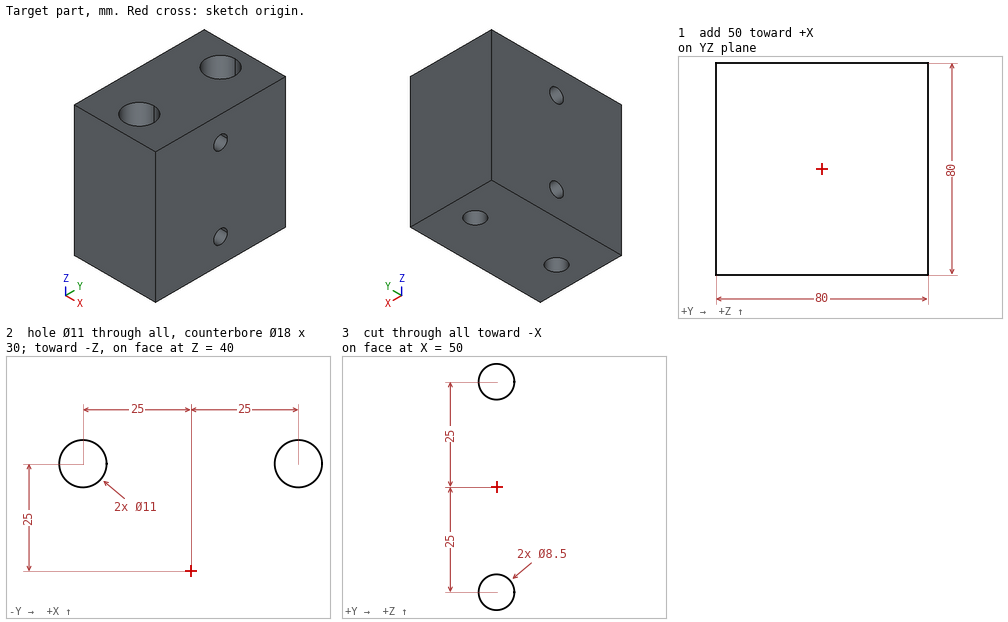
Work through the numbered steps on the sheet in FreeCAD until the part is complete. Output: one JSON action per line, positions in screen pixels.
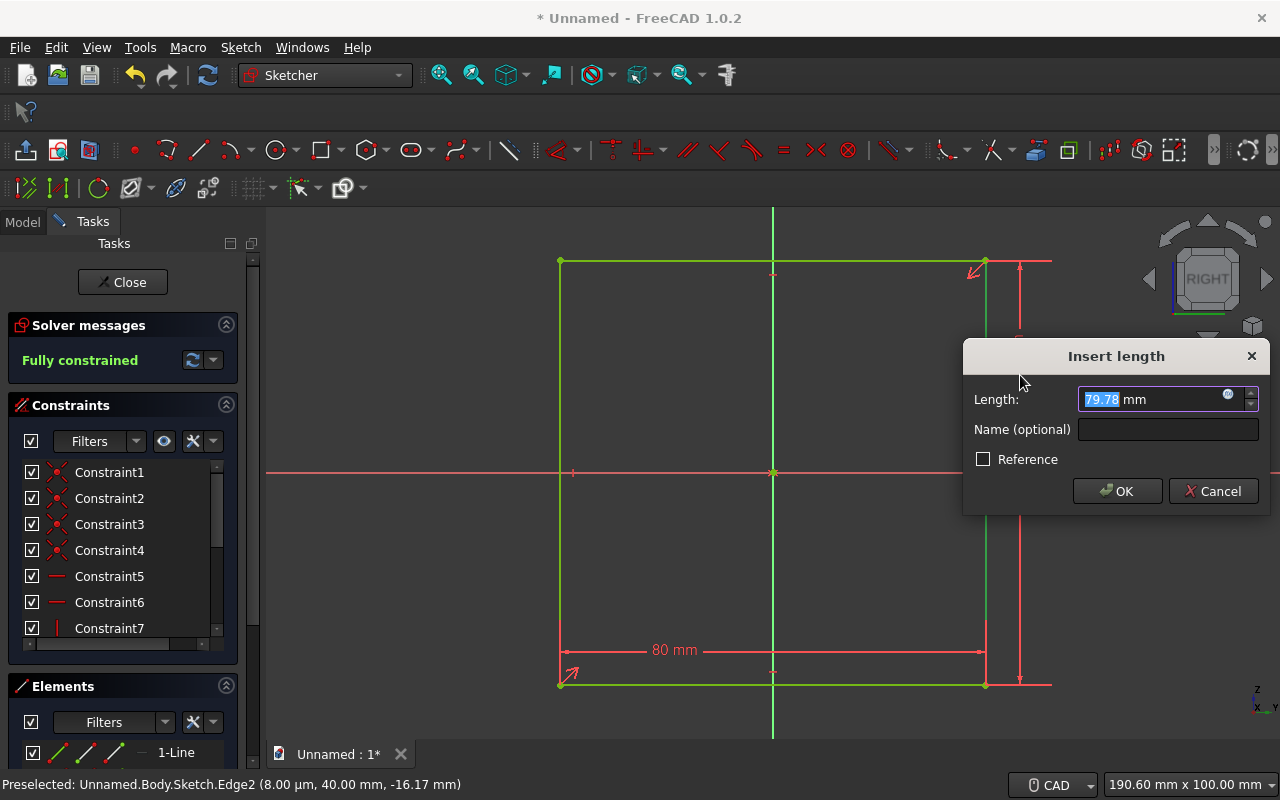
{"action": "type", "text": "80"}
{"action": "key", "text": "Return"}
{"action": "key", "text": "Escape"}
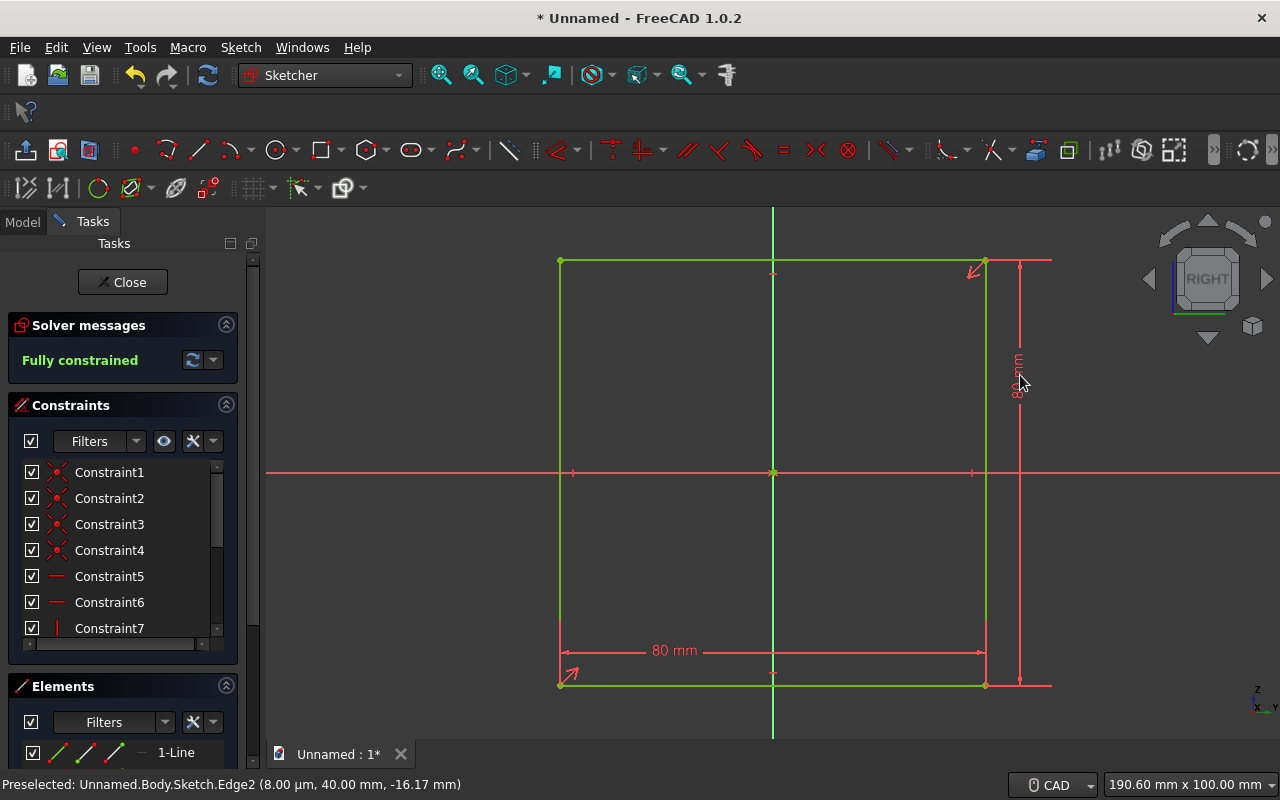
{"action": "left_click", "coordinate": [123, 282]}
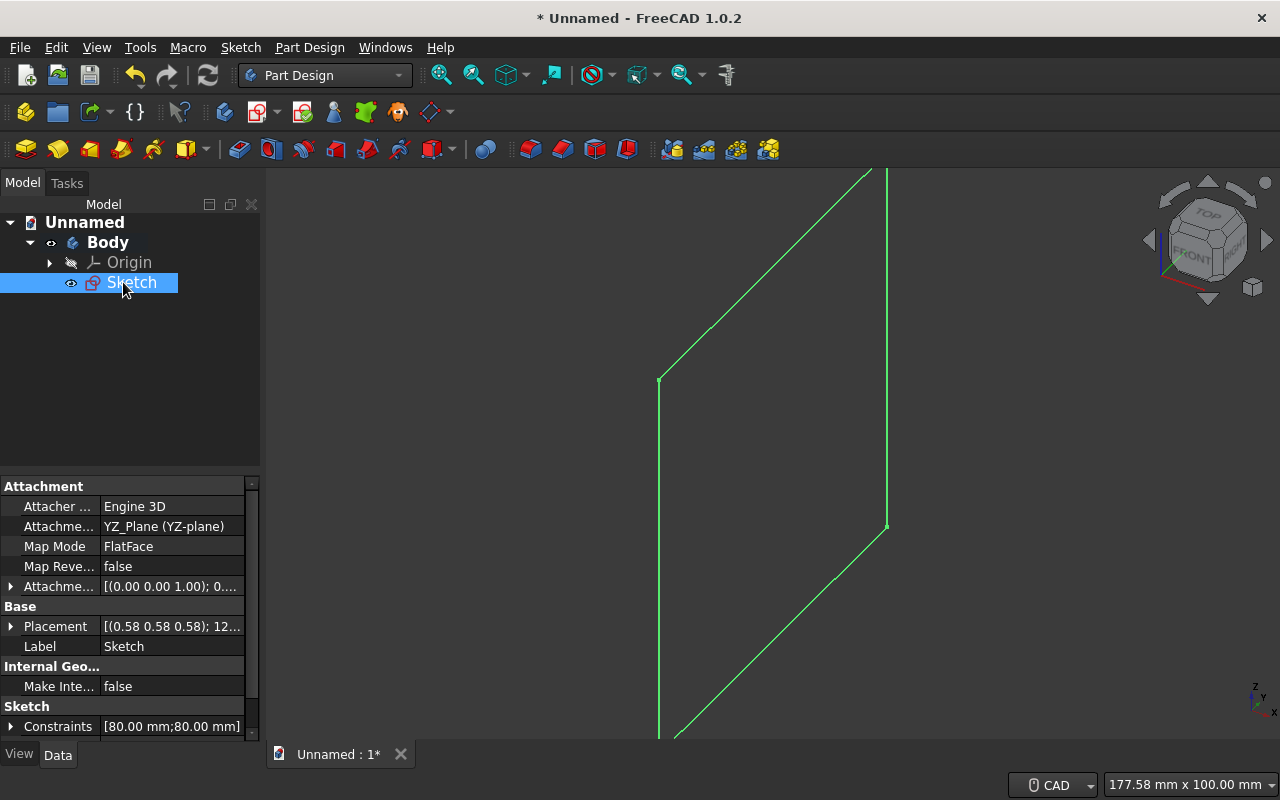
{"action": "left_click", "coordinate": [26, 150]}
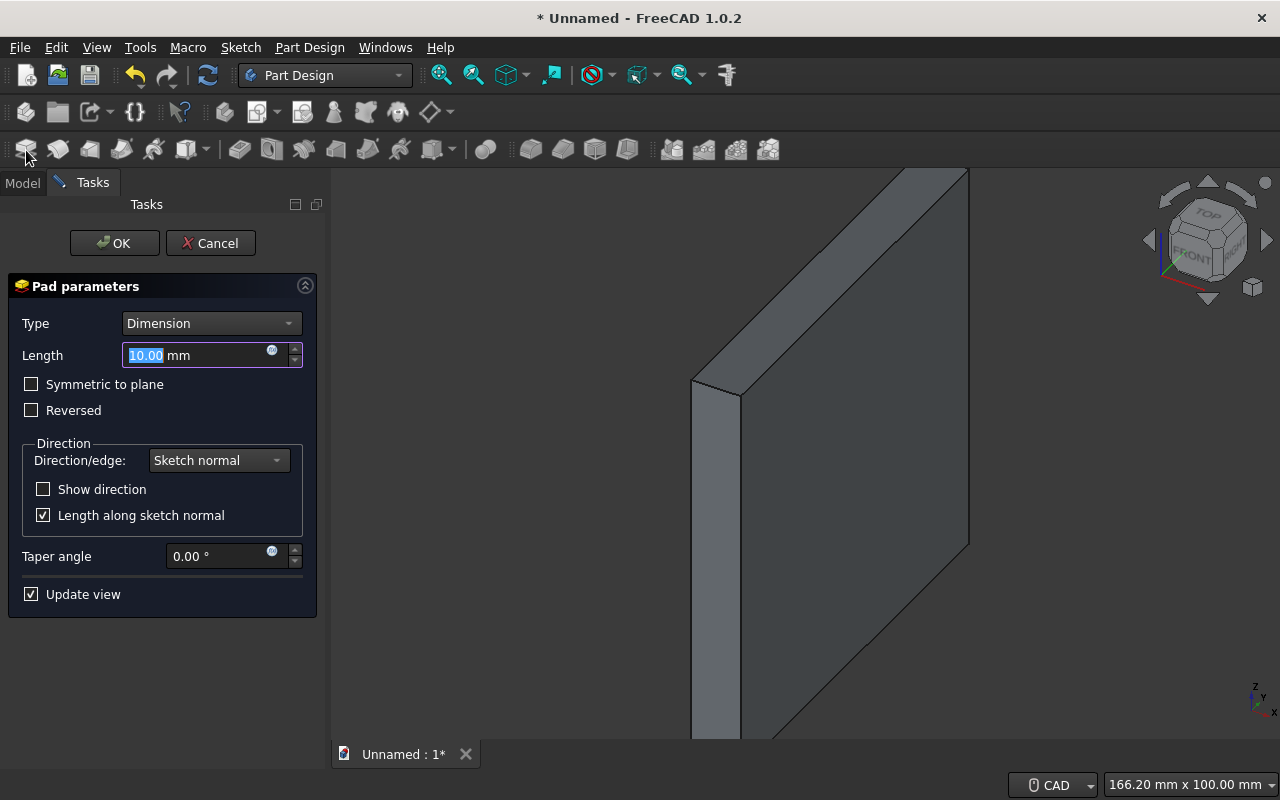
{"action": "type", "text": "50"}
{"action": "key", "text": "Tab"}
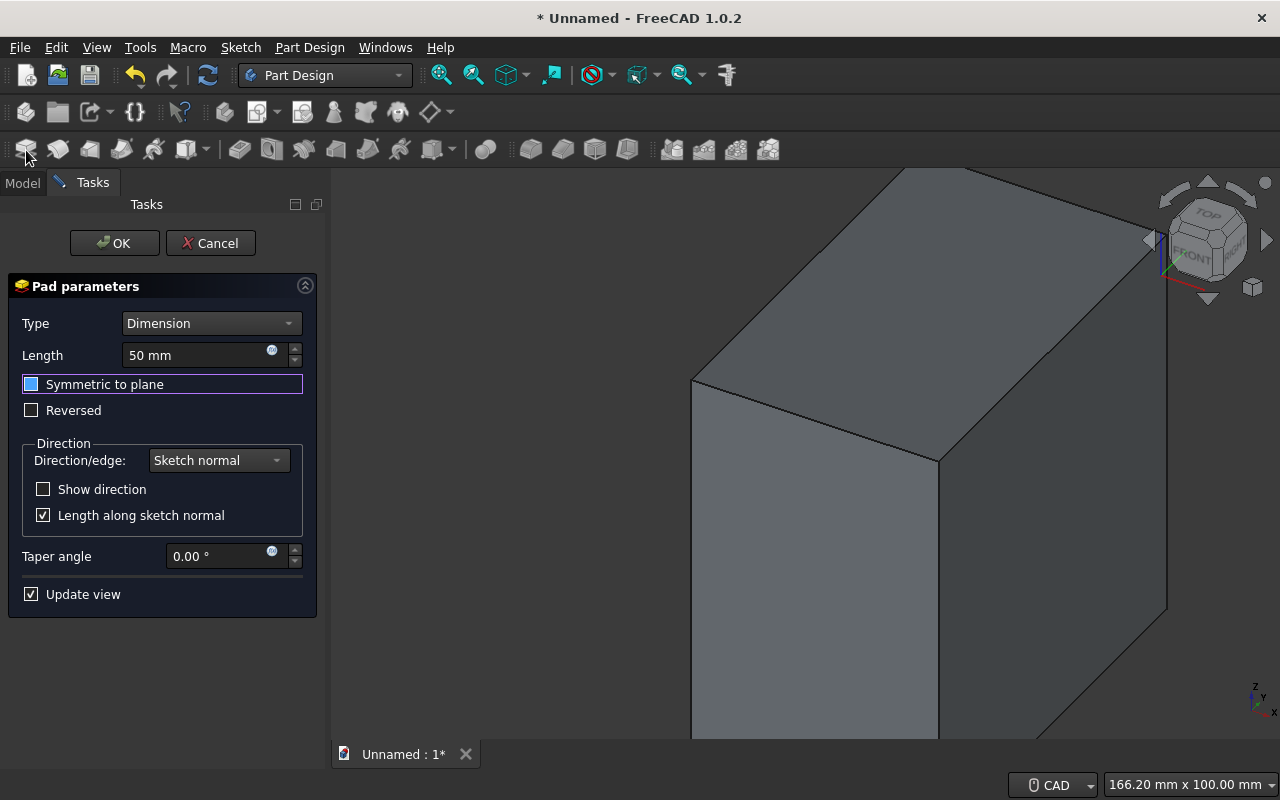
{"action": "left_click", "coordinate": [115, 243]}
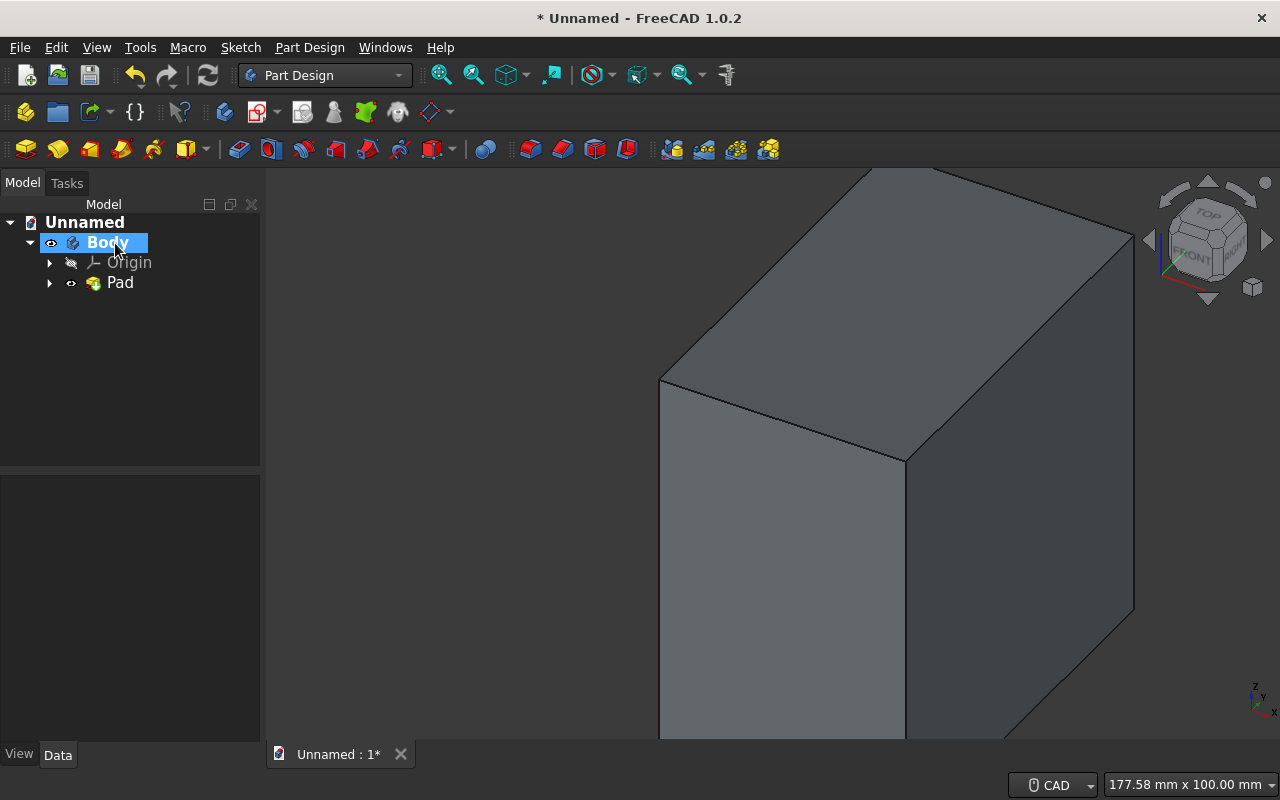
{"action": "left_click", "coordinate": [442, 76]}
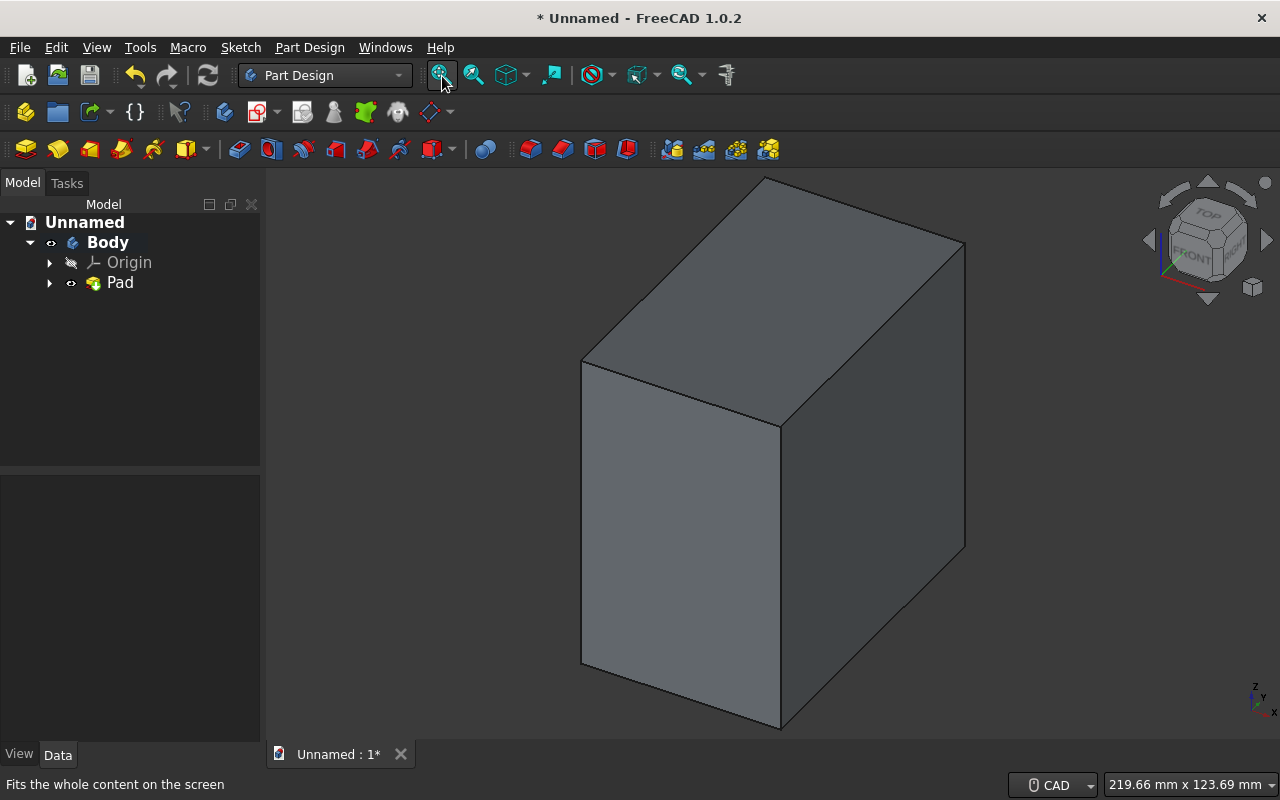
{"action": "left_click", "coordinate": [799, 275]}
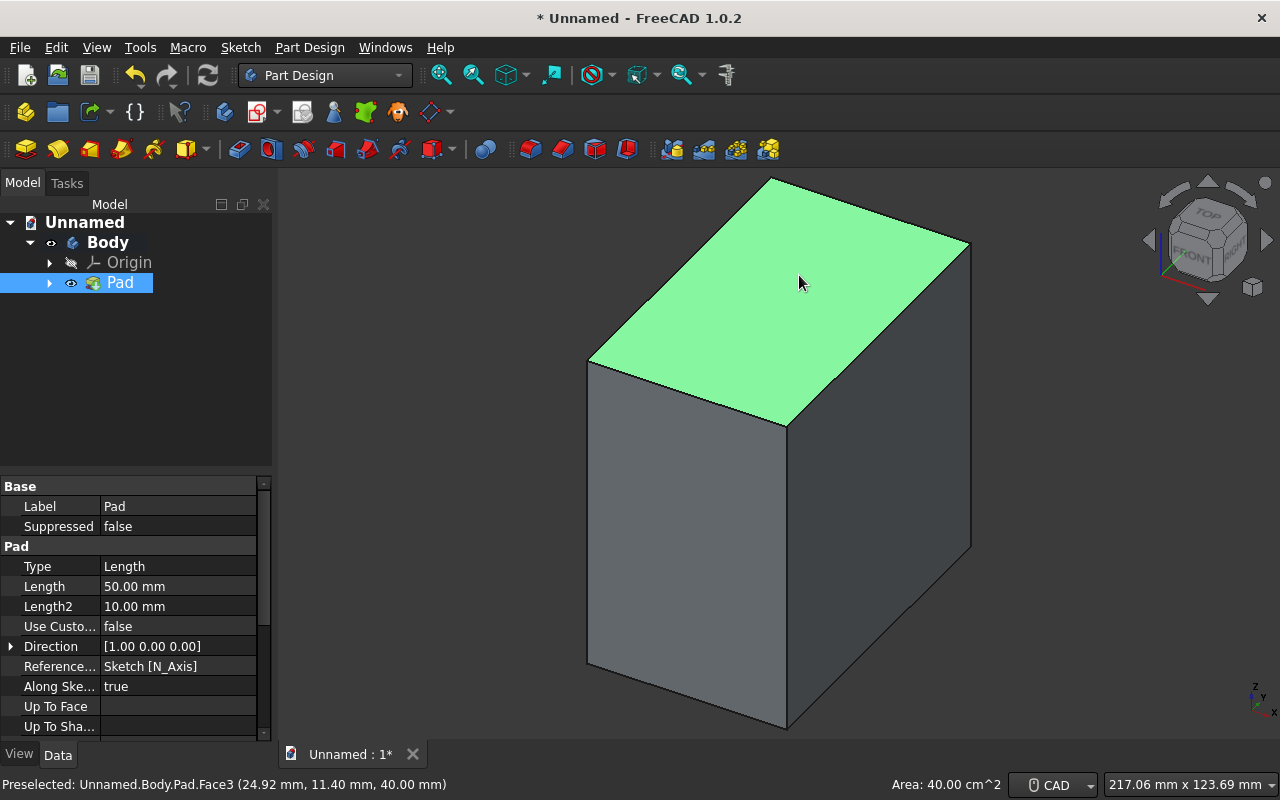
{"action": "left_click", "coordinate": [258, 112]}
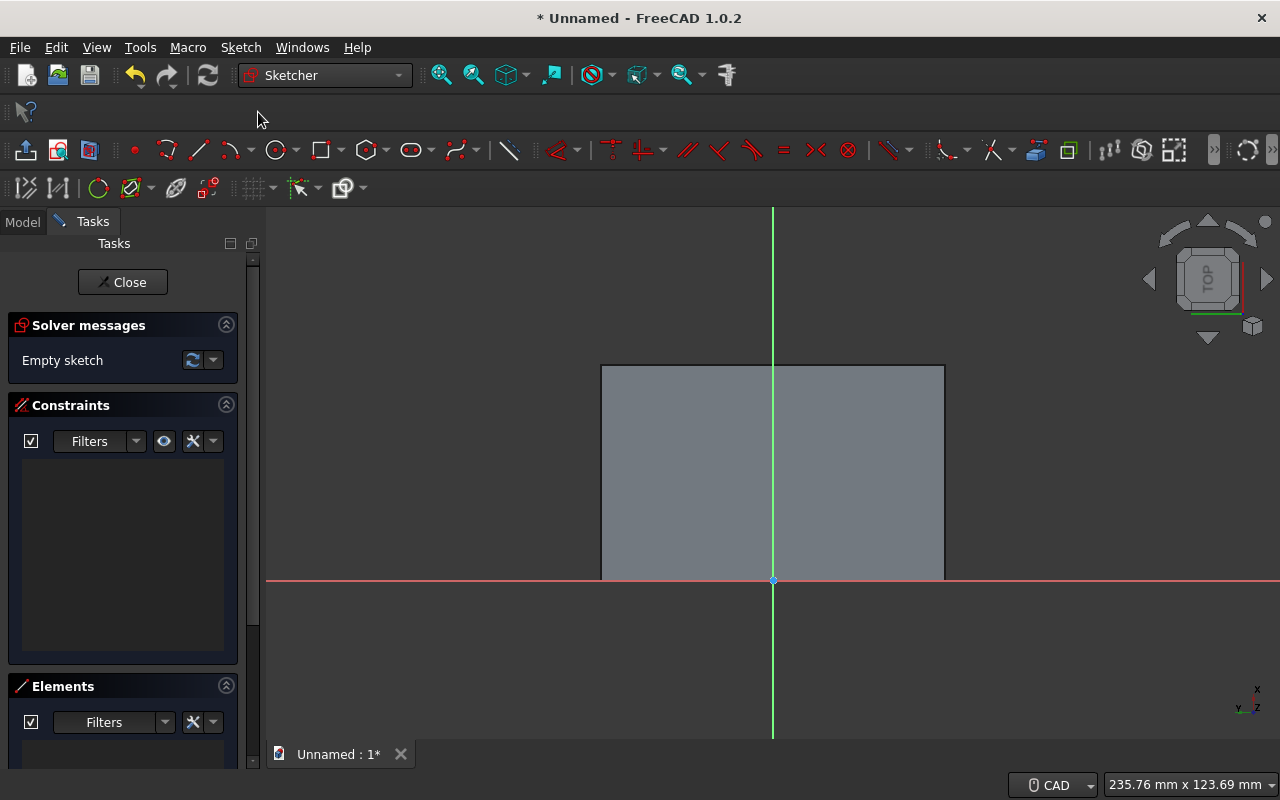
{"action": "scroll", "coordinate": [829, 549], "scroll_direction": "up", "scroll_amount": 4}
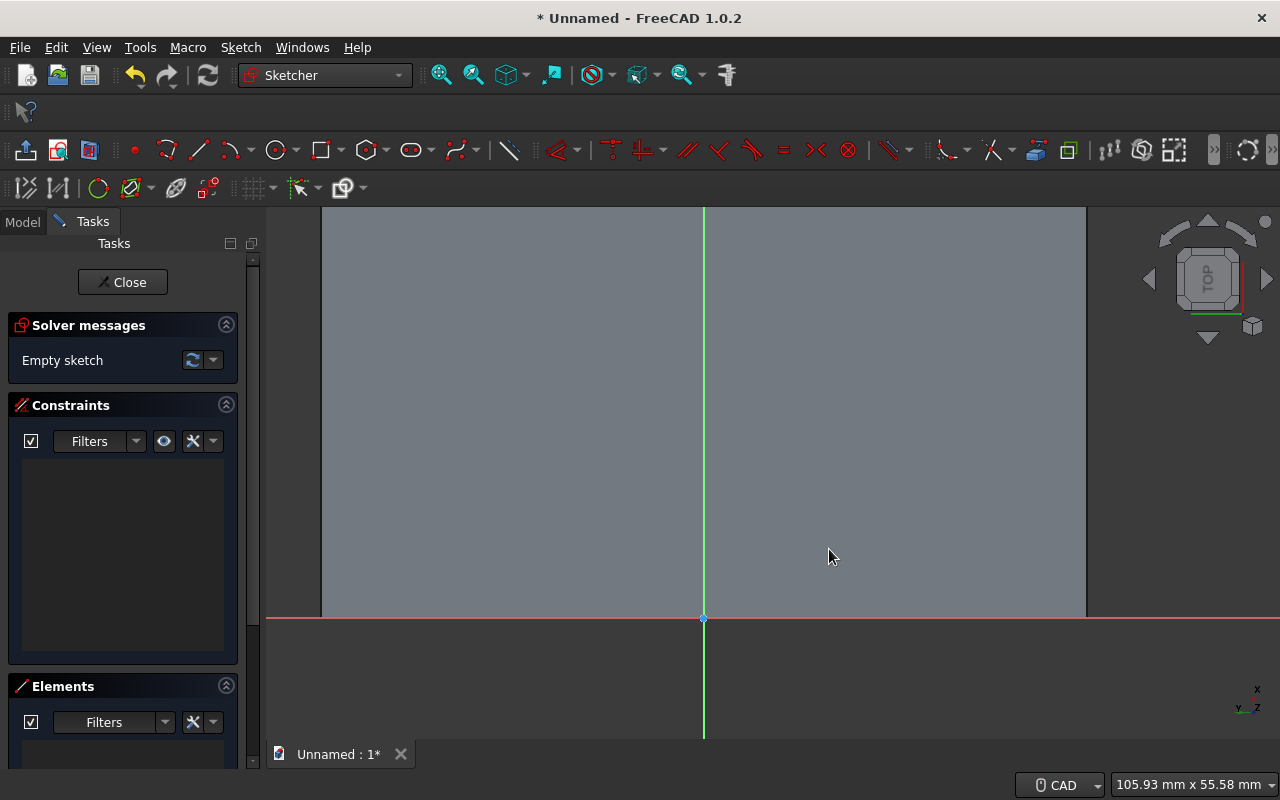
{"action": "left_click", "coordinate": [276, 150]}